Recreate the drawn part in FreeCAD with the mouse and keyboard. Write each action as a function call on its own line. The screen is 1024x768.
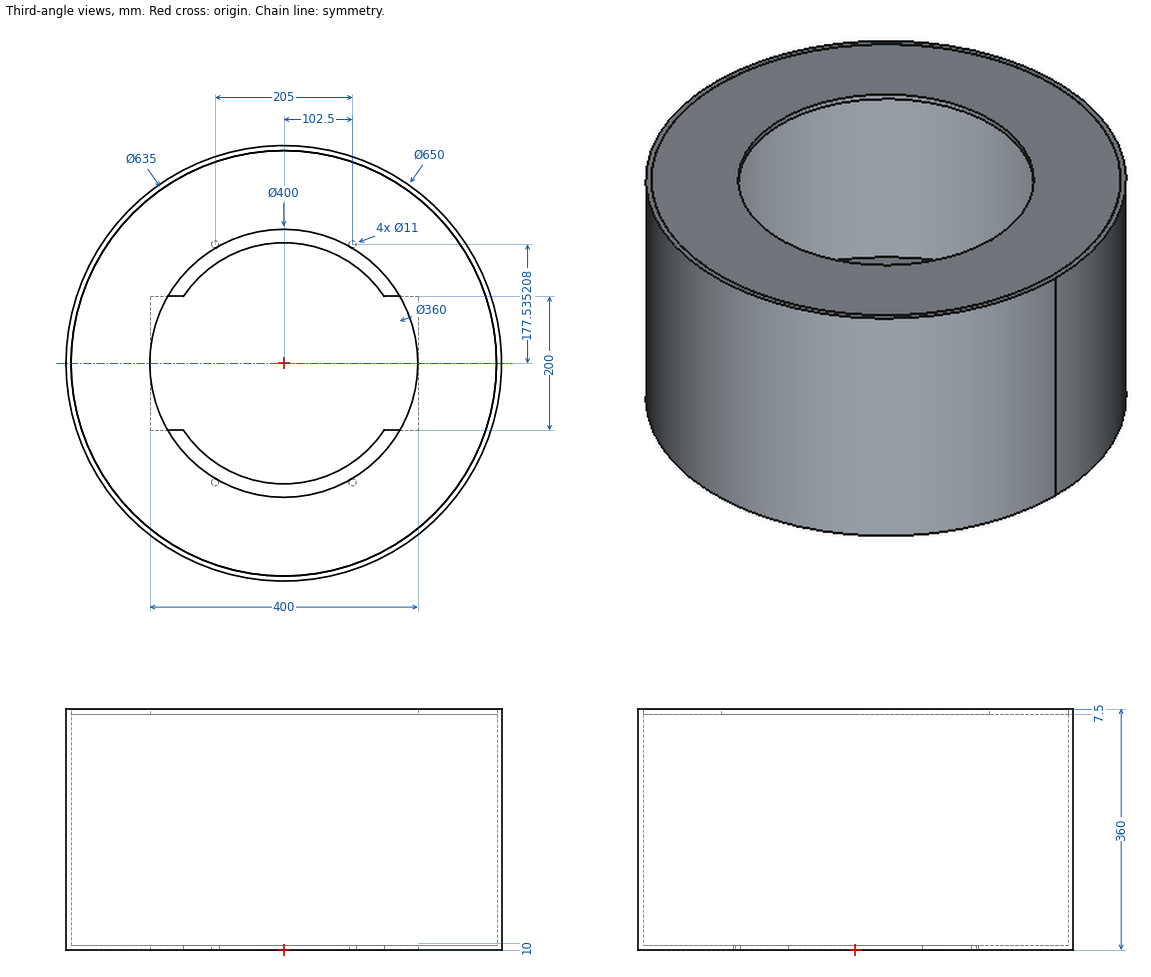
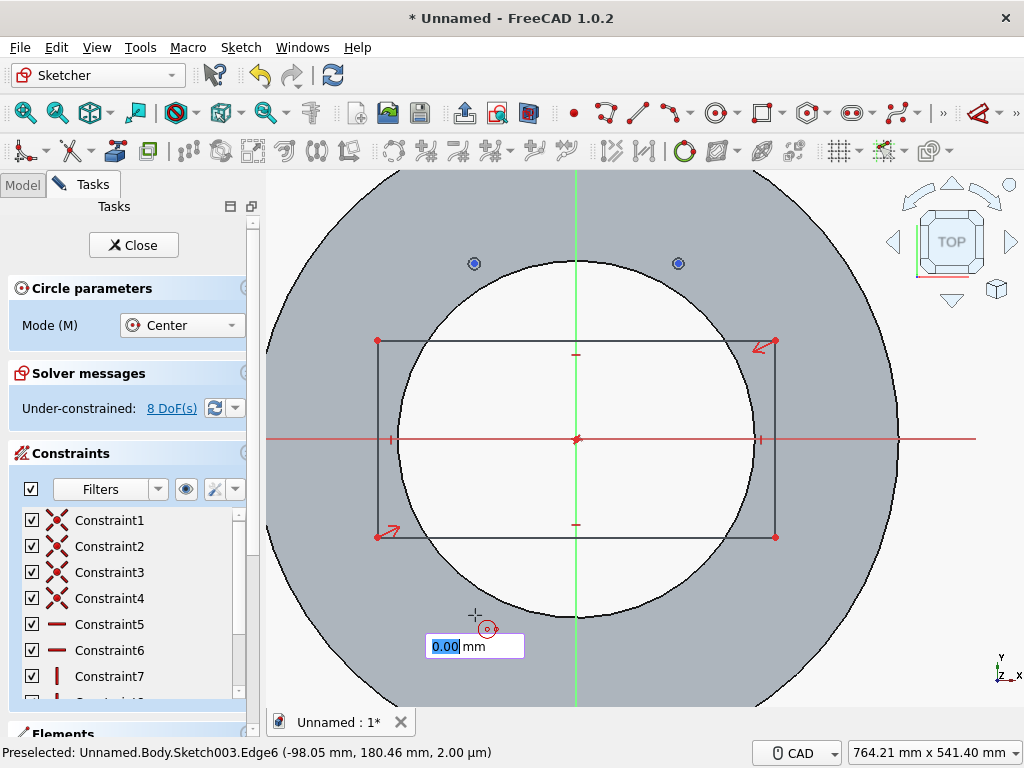
scroll(479, 612, up, 6)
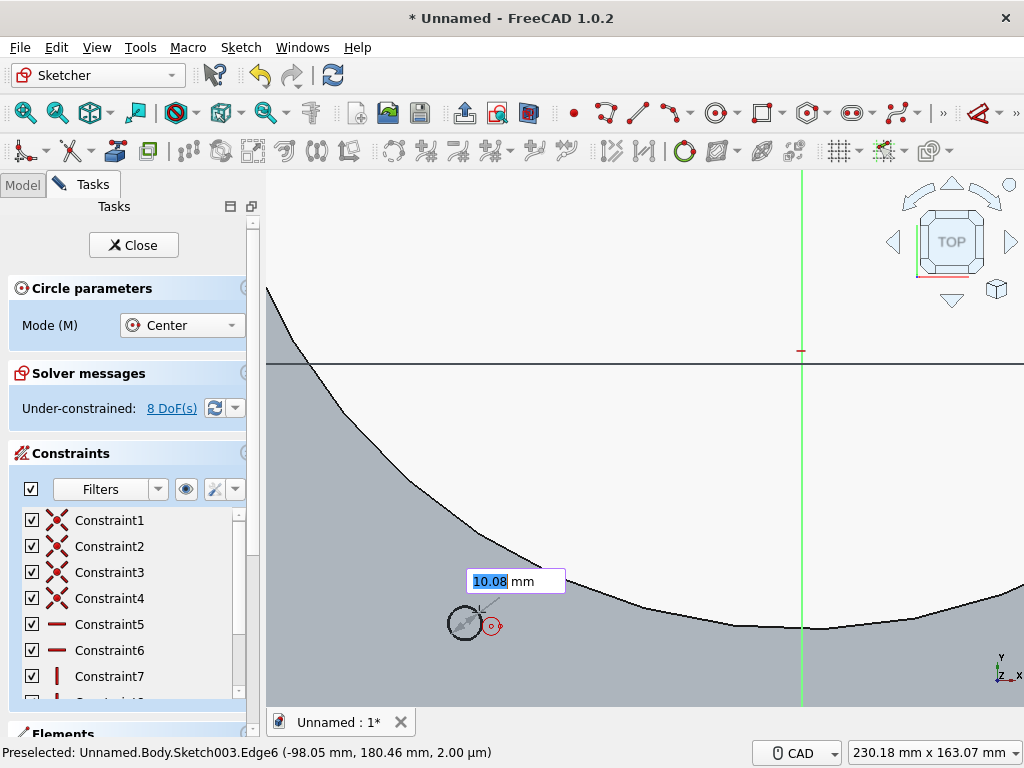
click(477, 609)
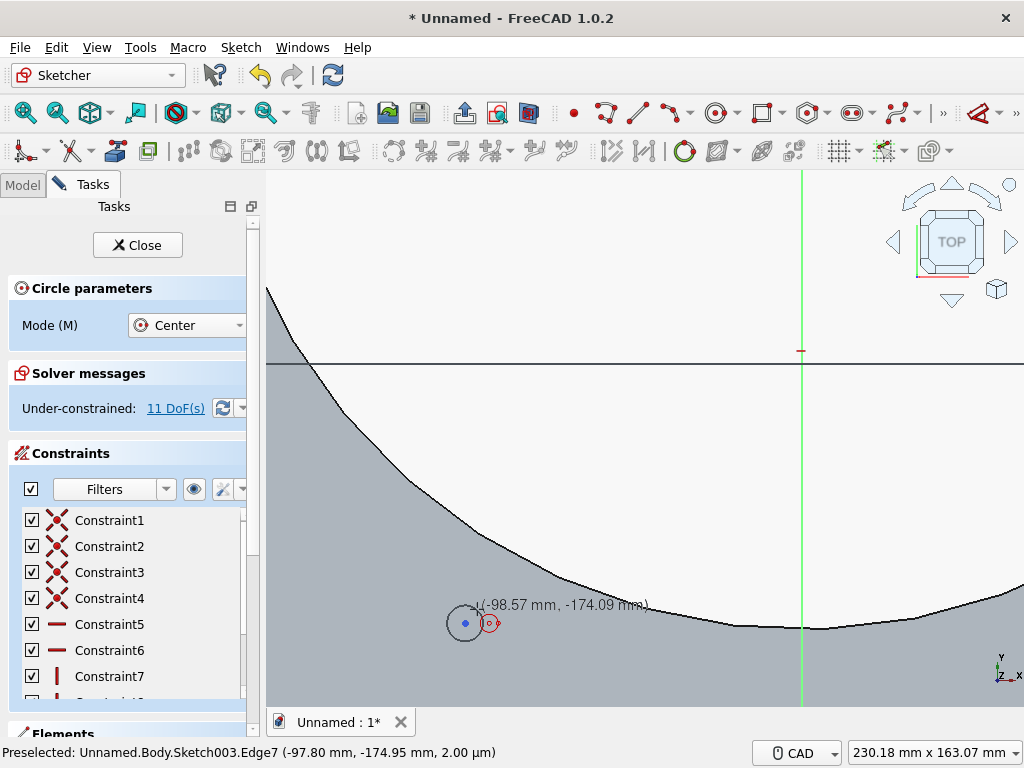
scroll(479, 612, down, 6)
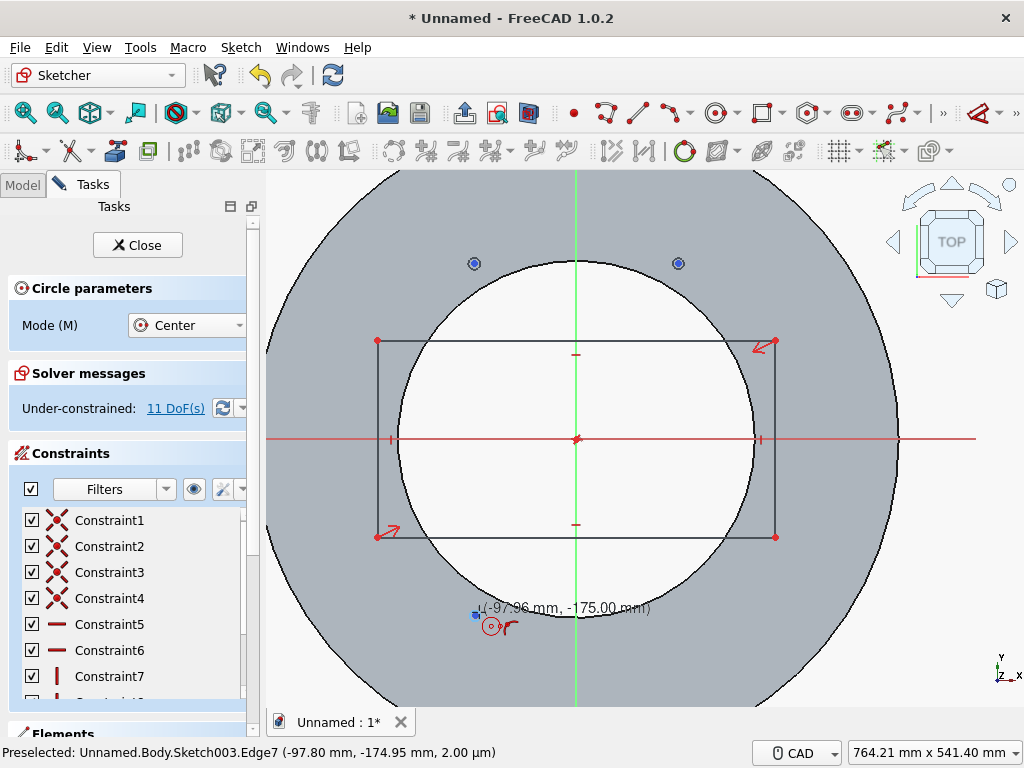
scroll(678, 615, up, 8)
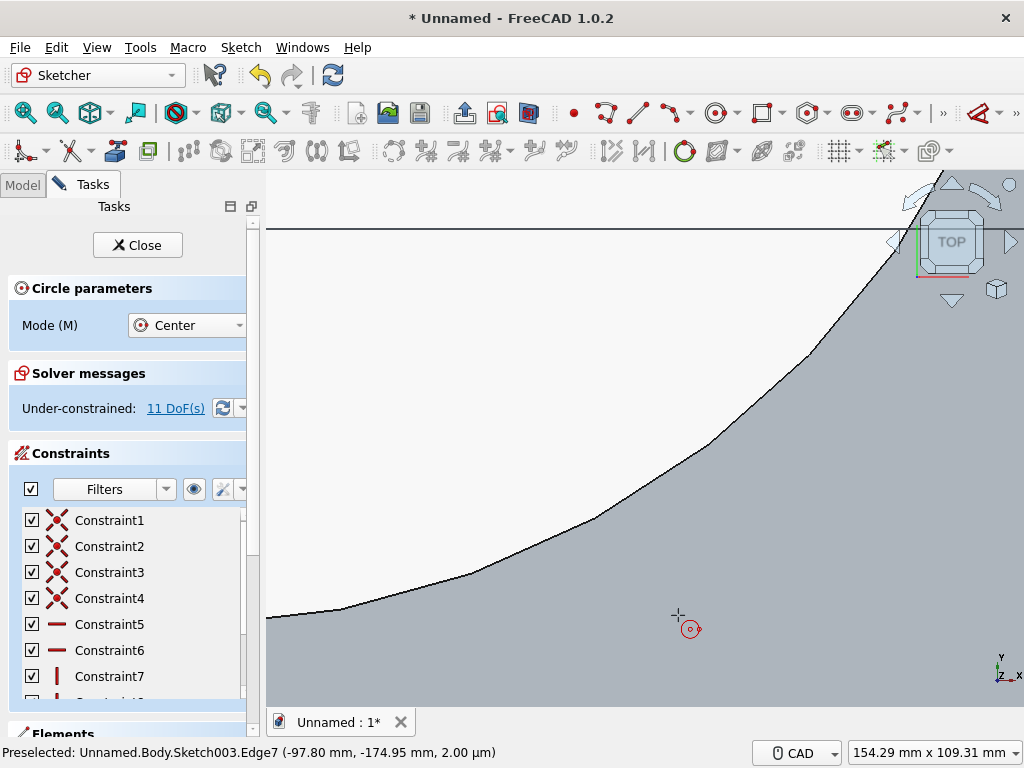
scroll(679, 615, down, 8)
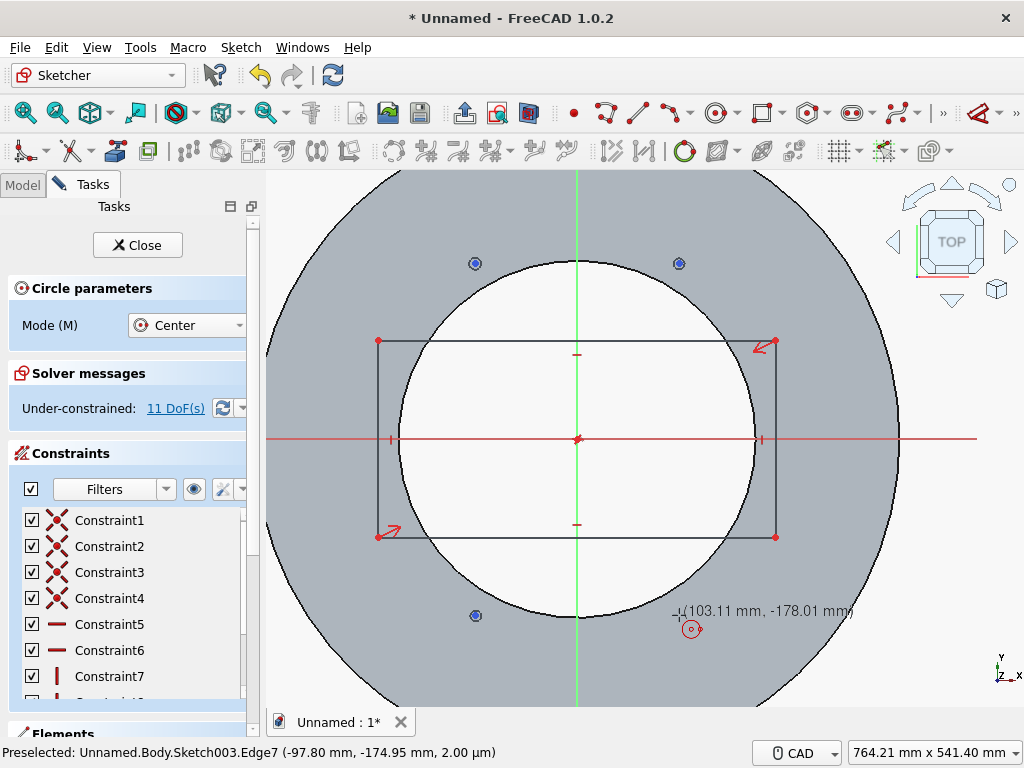
click(679, 615)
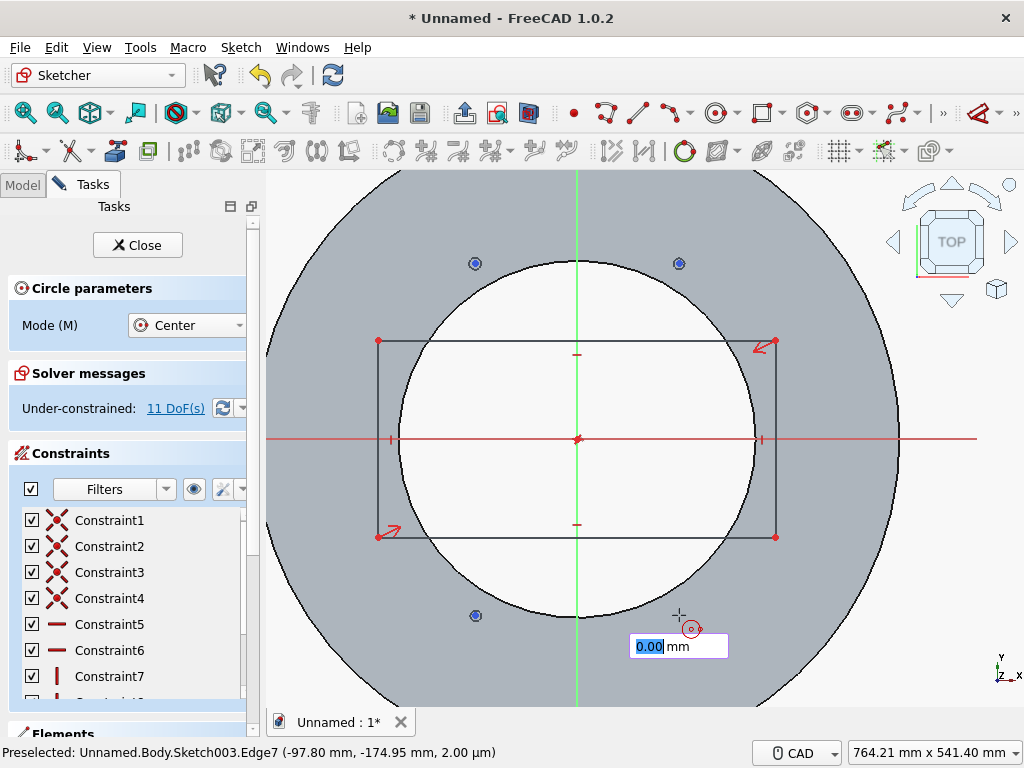
scroll(683, 612, up, 6)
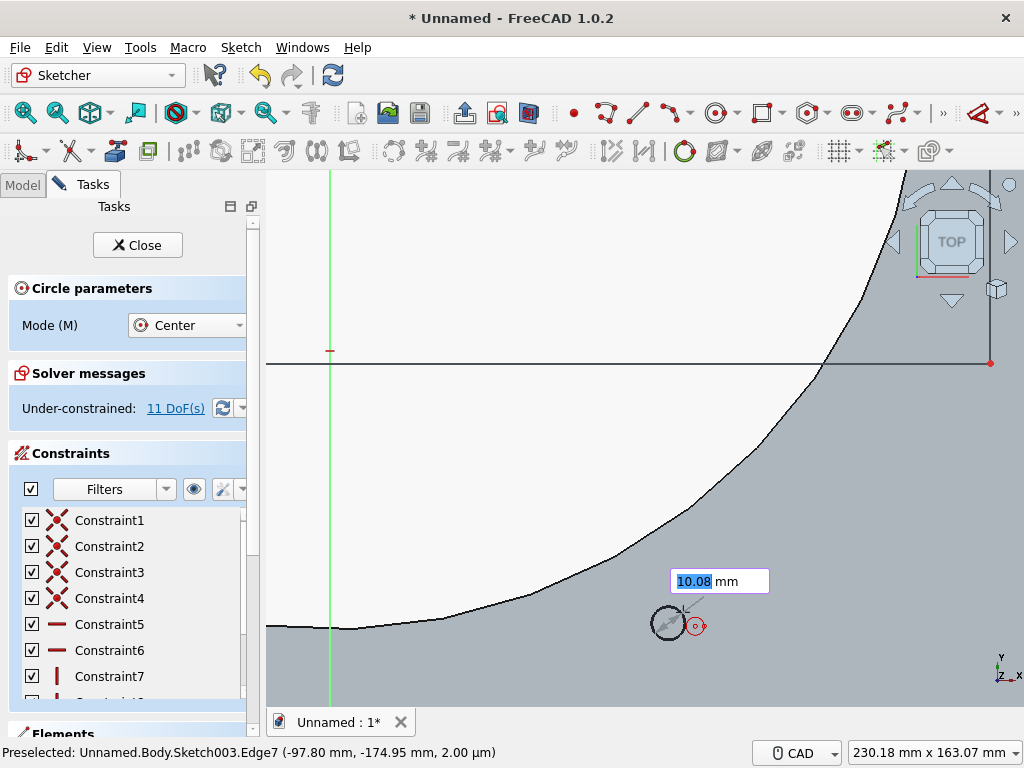
click(681, 609)
key(Escape)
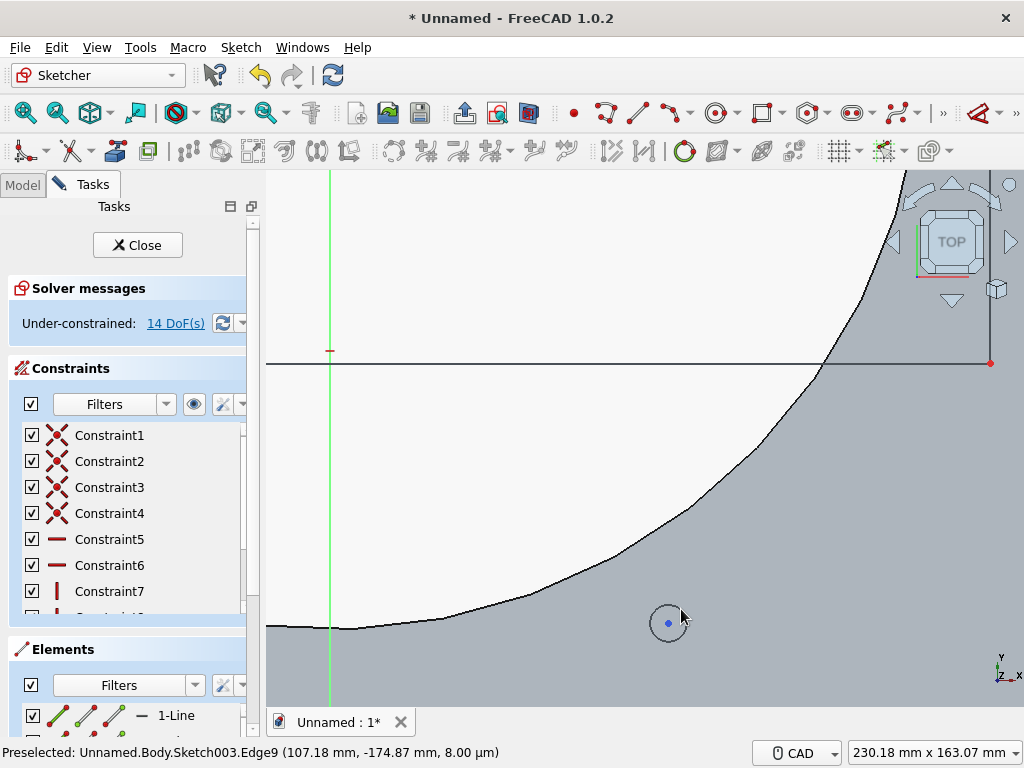
scroll(683, 612, down, 6)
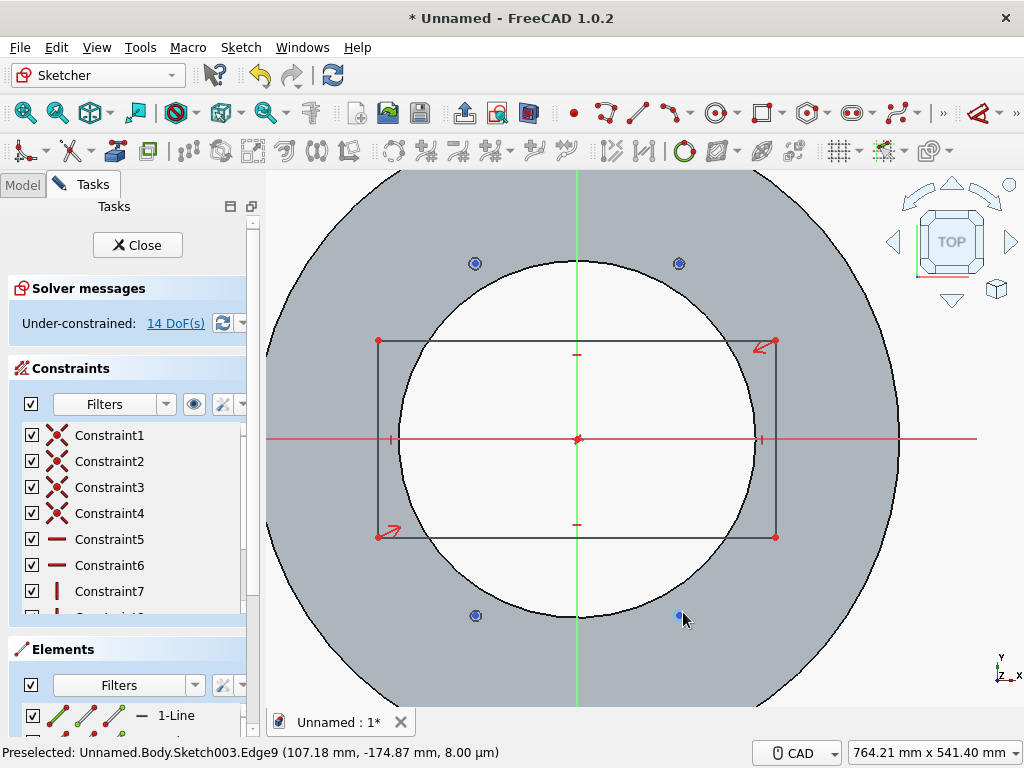
scroll(683, 260, up, 5)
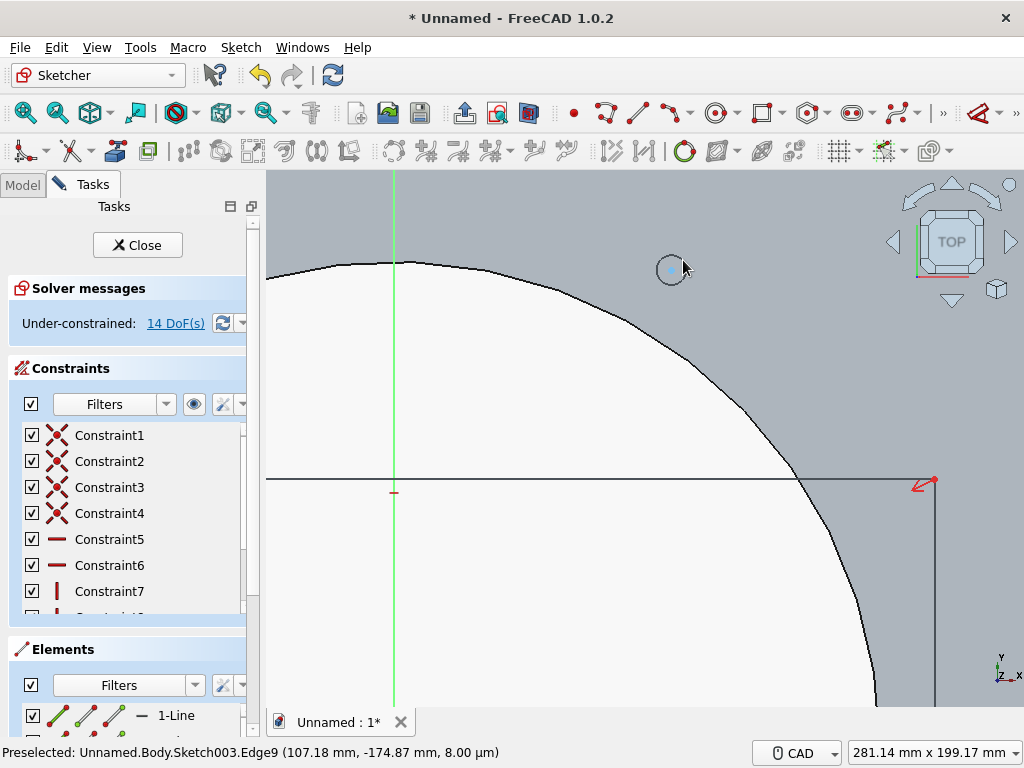
click(682, 260)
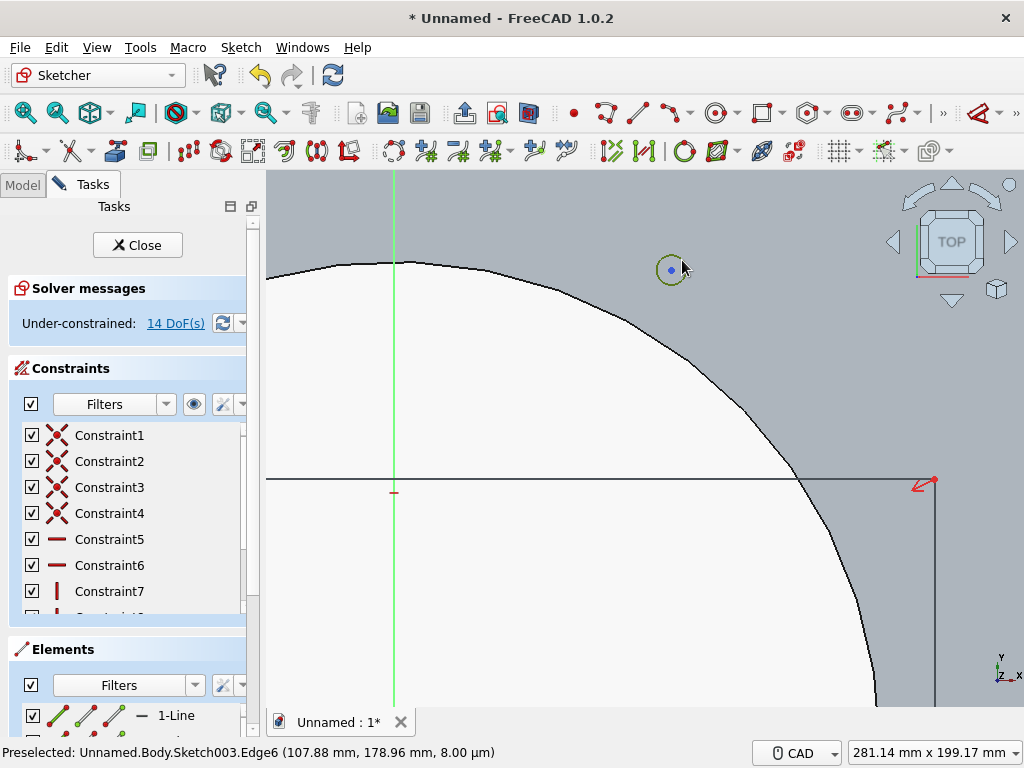
scroll(683, 259, down, 5)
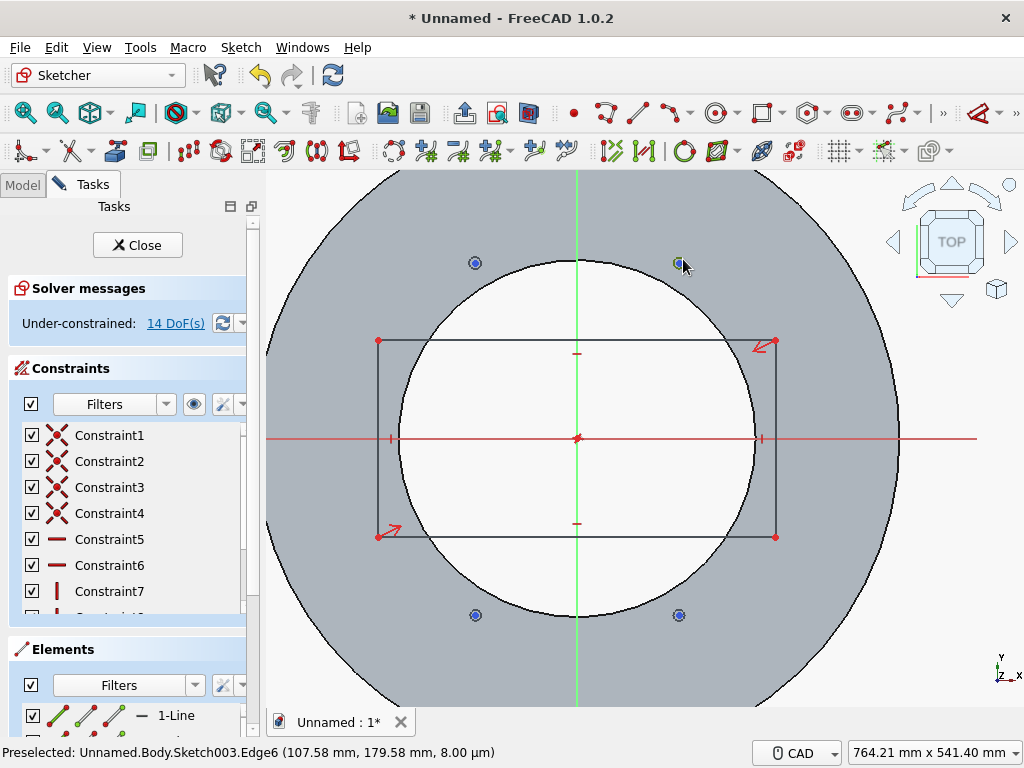
scroll(479, 259, up, 5)